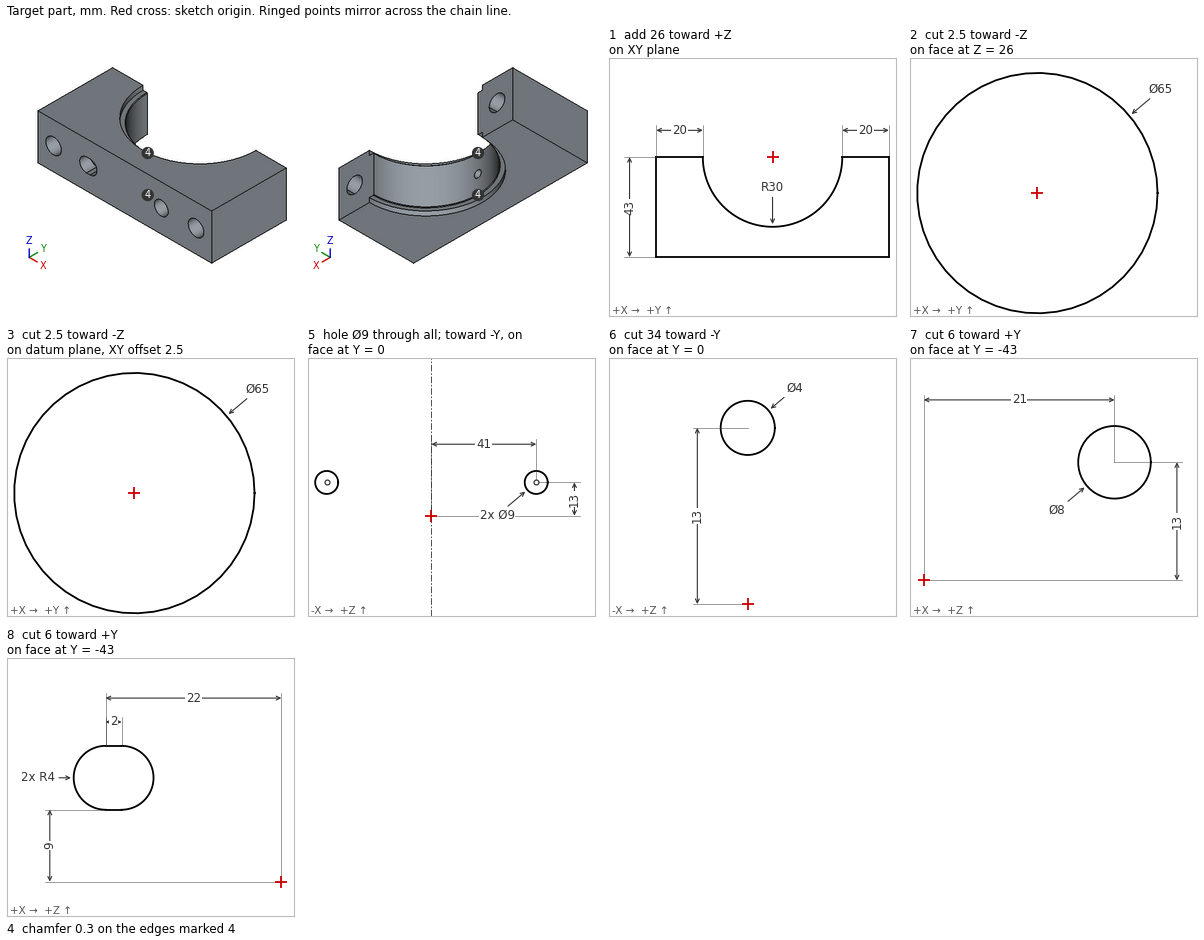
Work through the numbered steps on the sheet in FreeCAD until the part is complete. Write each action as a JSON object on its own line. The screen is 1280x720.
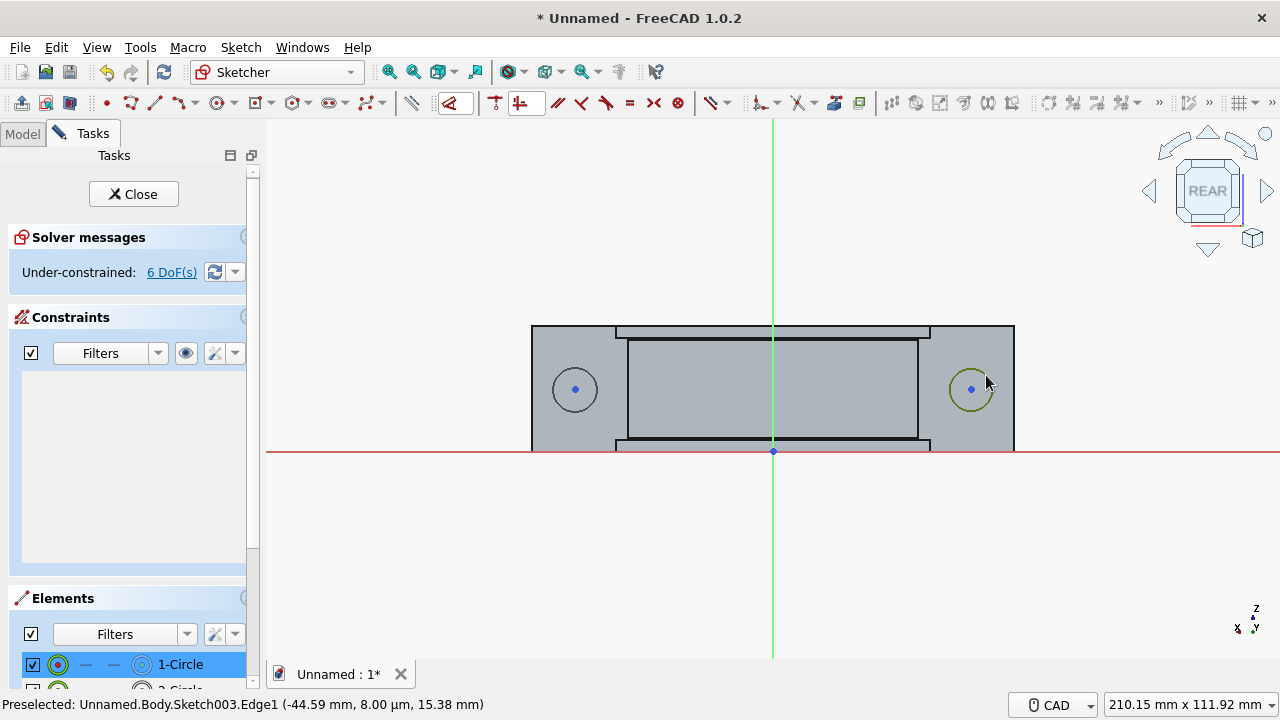
{"action": "left_click", "coordinate": [590, 374]}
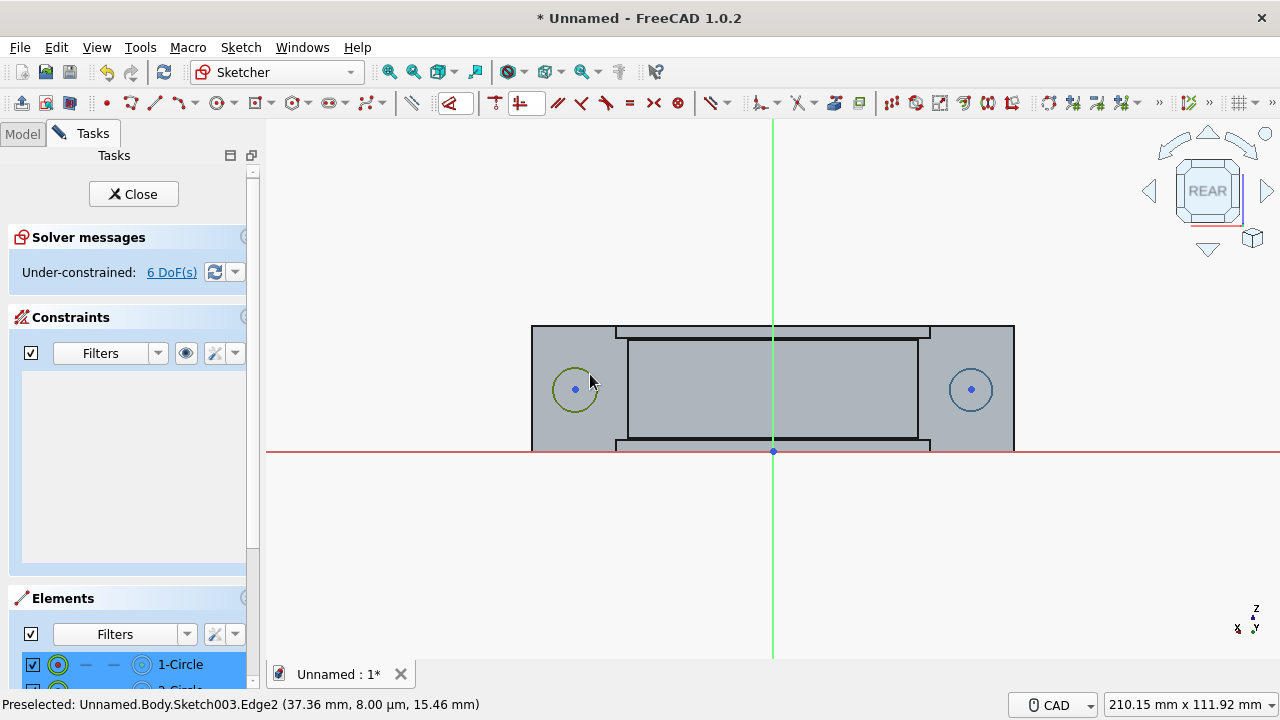
{"action": "left_click", "coordinate": [630, 104]}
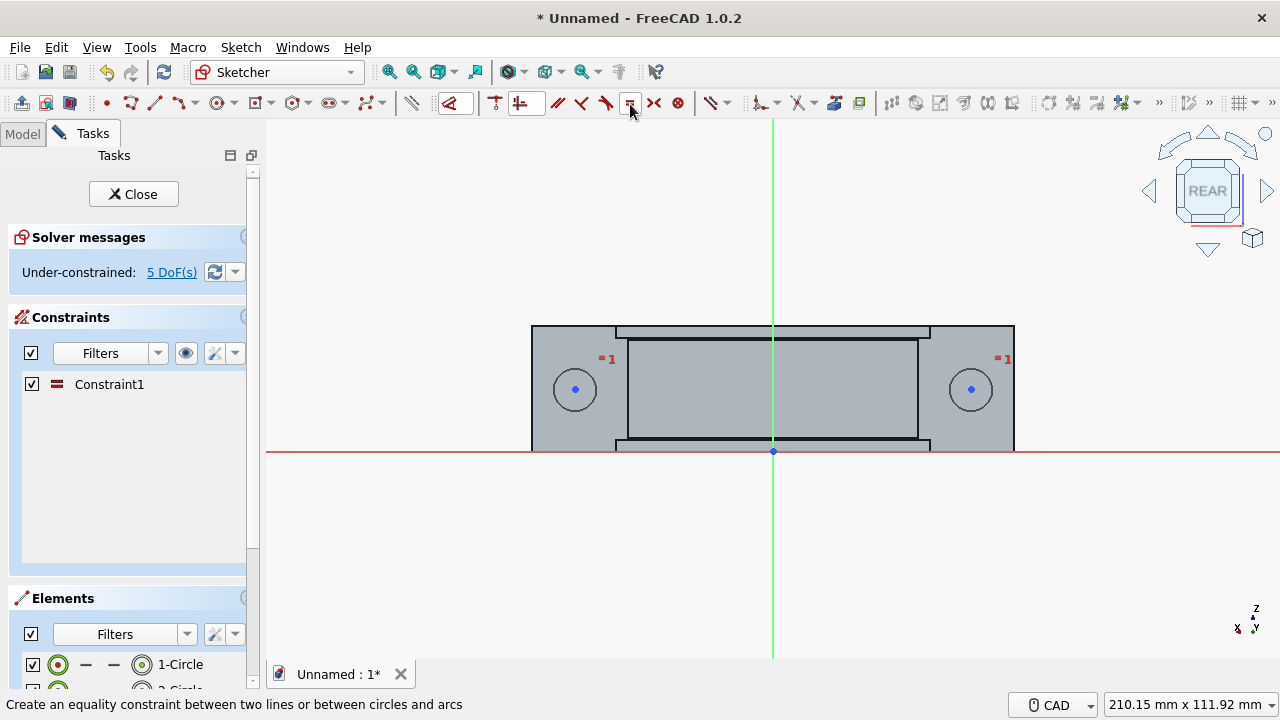
{"action": "left_click", "coordinate": [971, 390]}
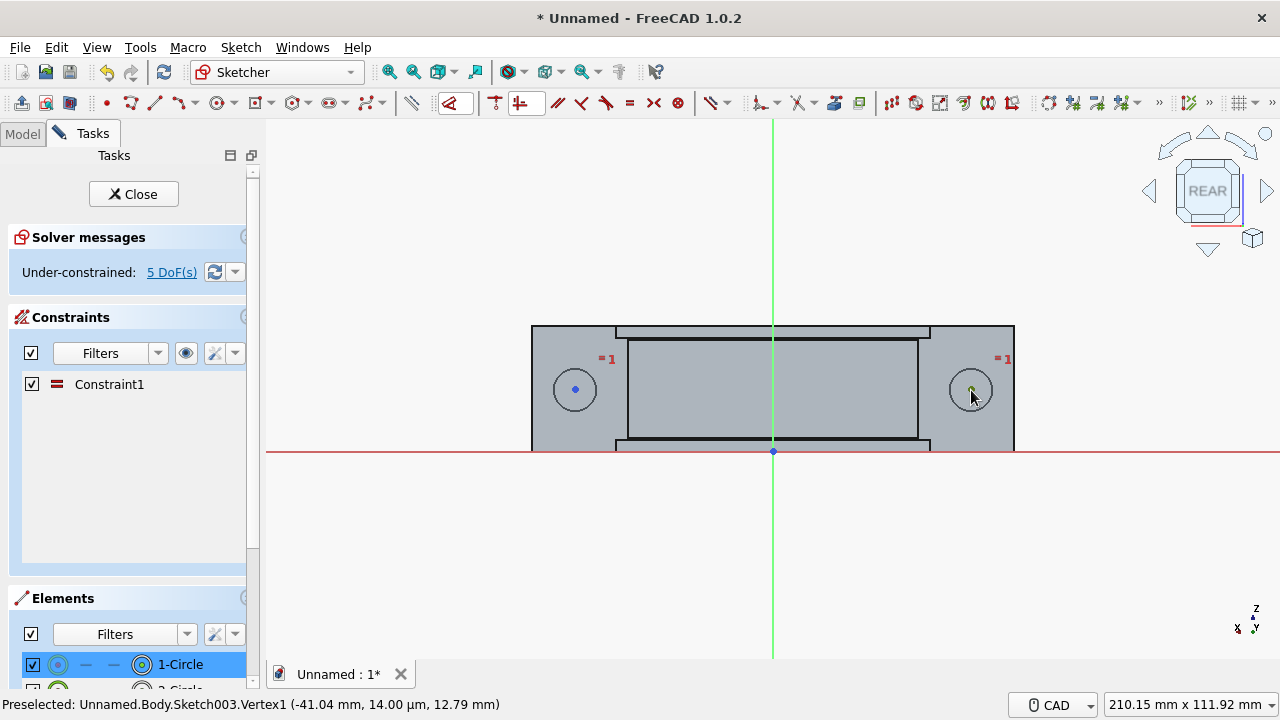
{"action": "left_click", "coordinate": [575, 390]}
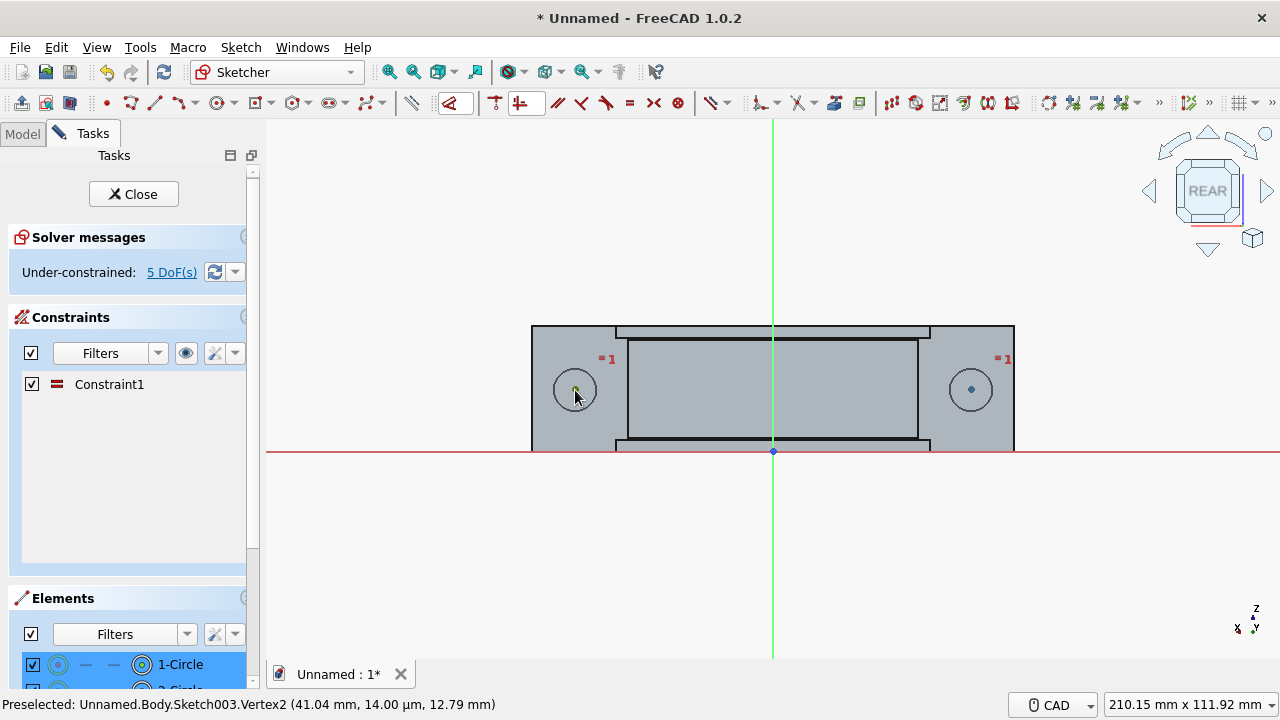
{"action": "left_click", "coordinate": [773, 596]}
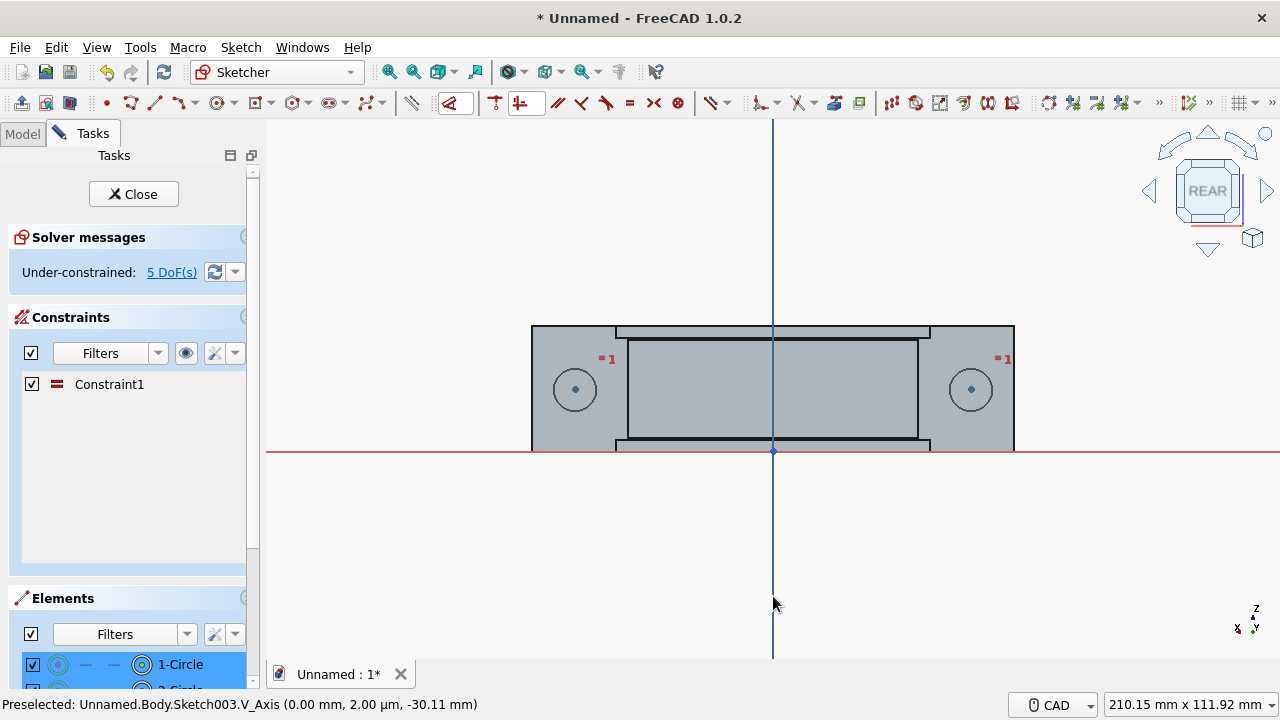
{"action": "left_click", "coordinate": [654, 104]}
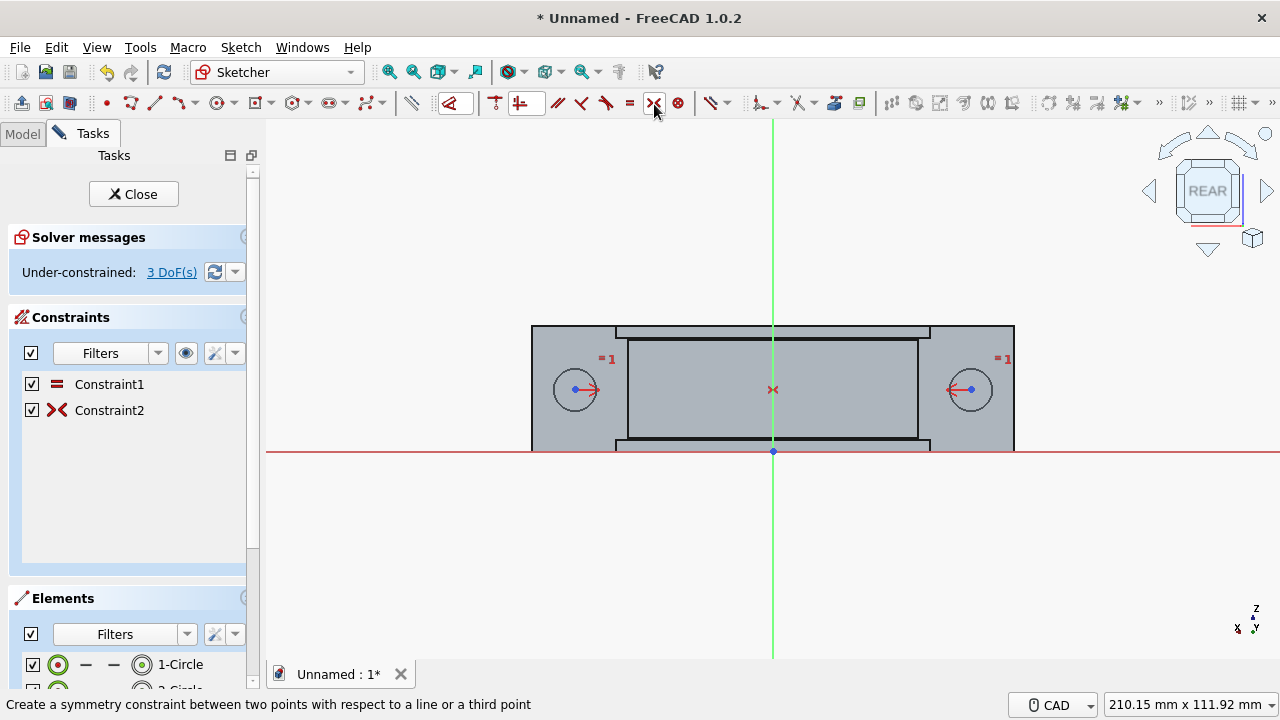
{"action": "left_click", "coordinate": [986, 375]}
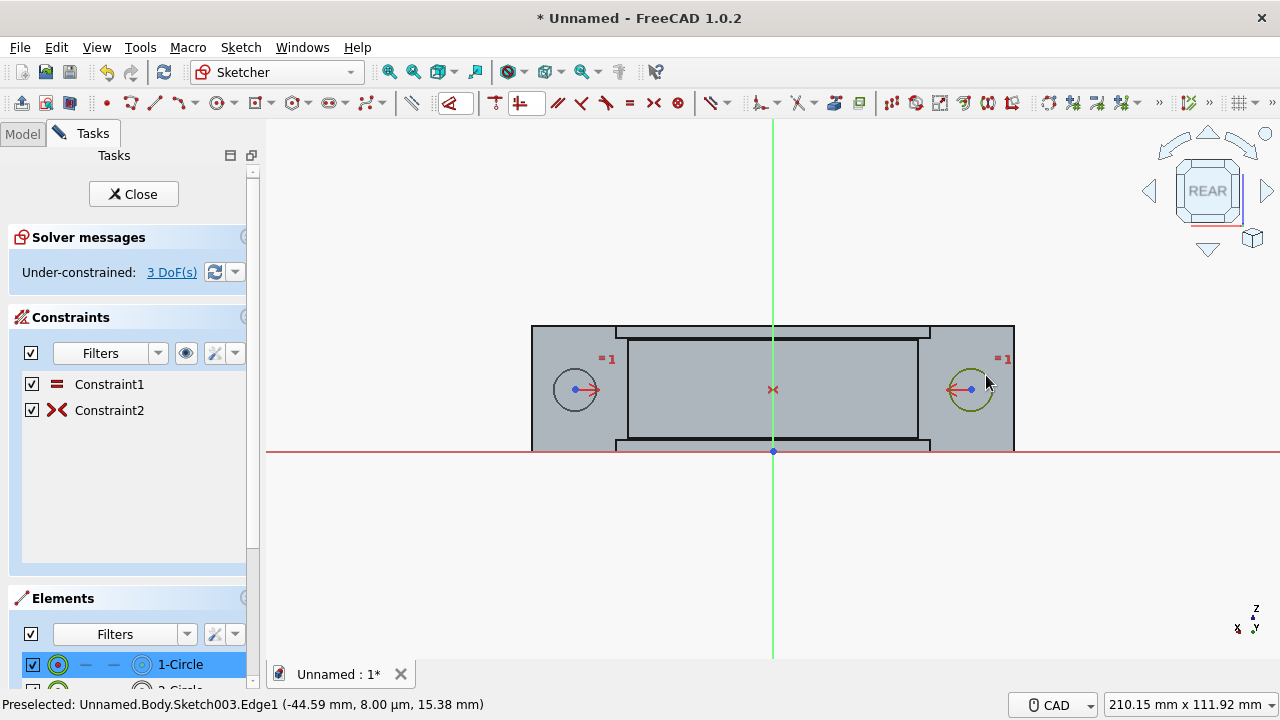
{"action": "key", "text": "k o"}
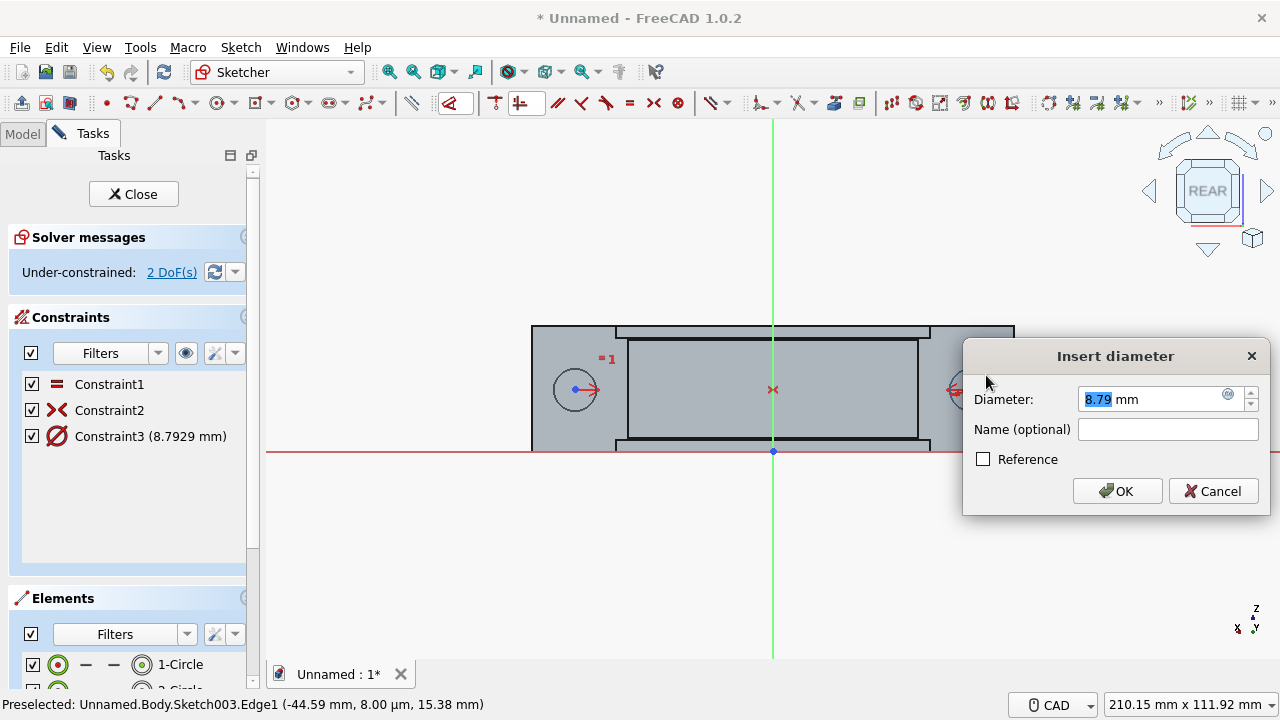
{"action": "type", "text": "9"}
{"action": "key", "text": "Return"}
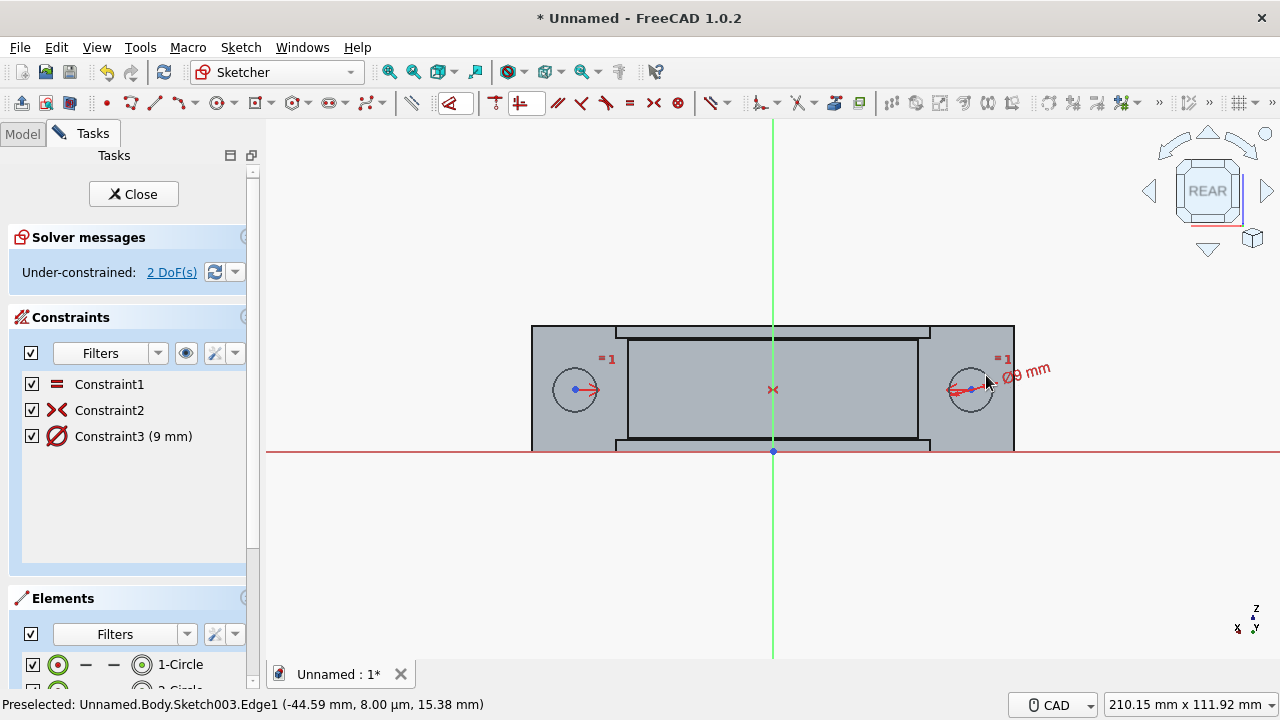
{"action": "left_click", "coordinate": [971, 390]}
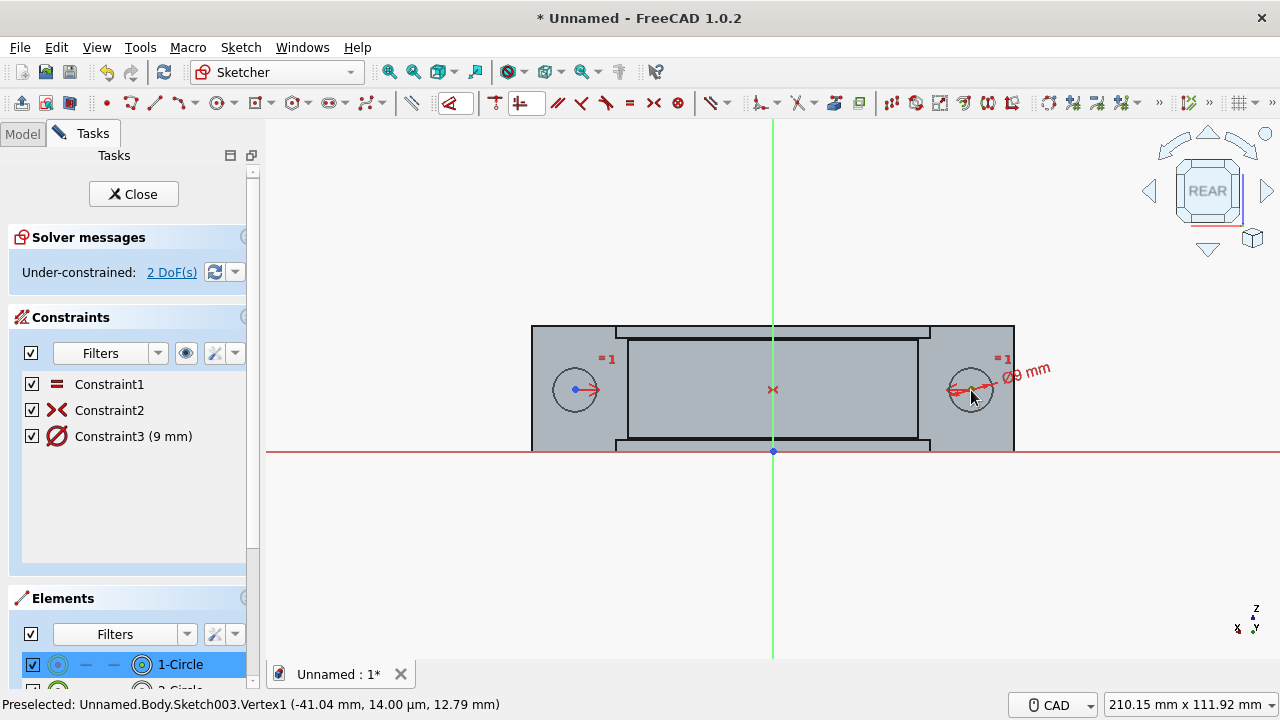
{"action": "left_click", "coordinate": [468, 104]}